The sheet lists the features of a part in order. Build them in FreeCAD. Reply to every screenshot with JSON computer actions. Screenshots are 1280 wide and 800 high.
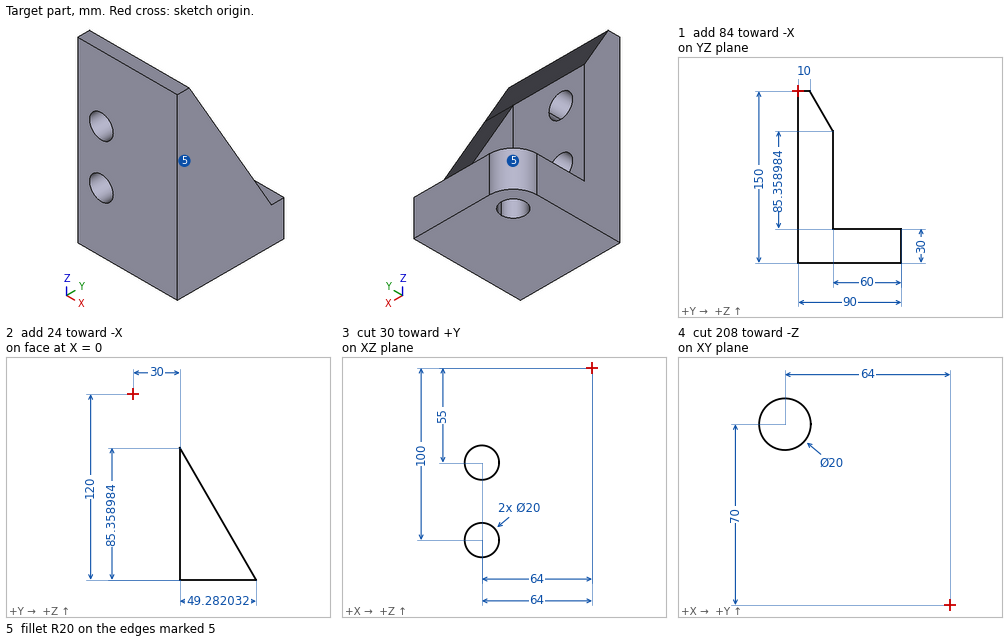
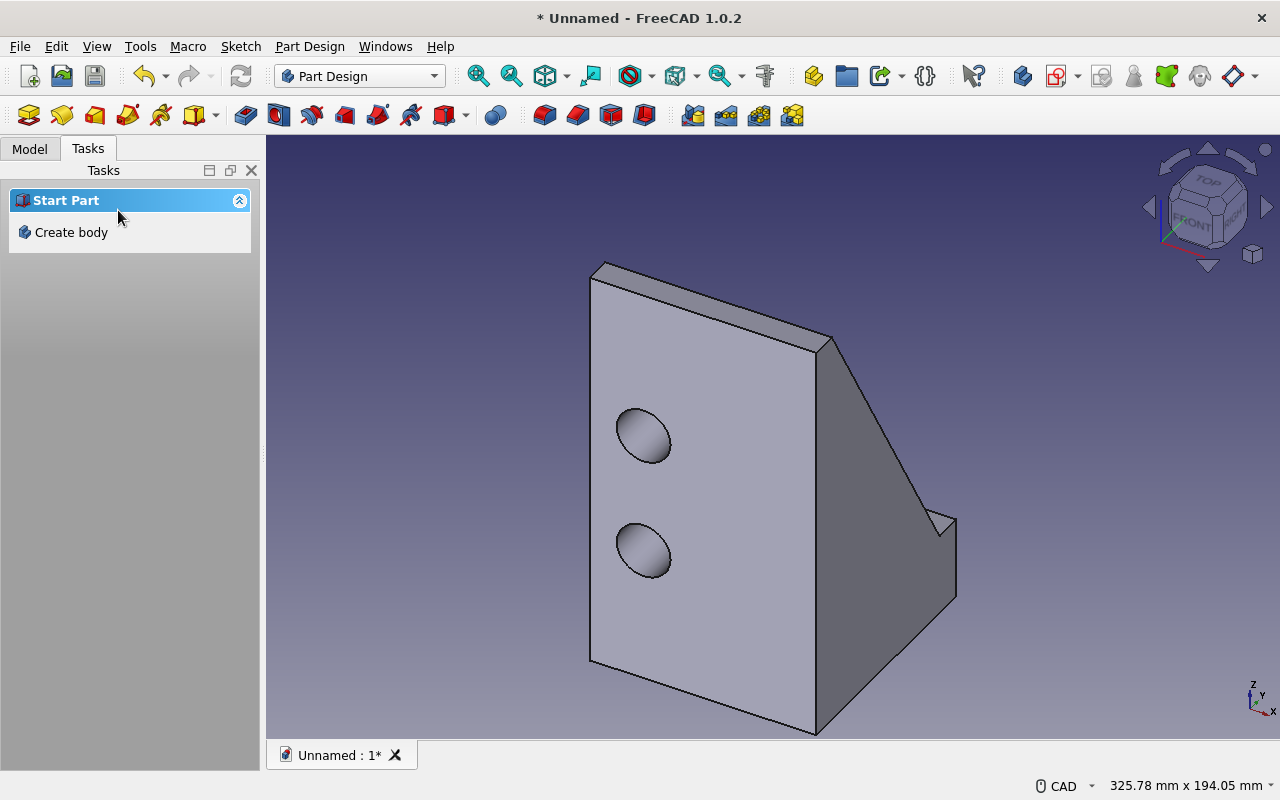
{"action": "key", "text": "0"}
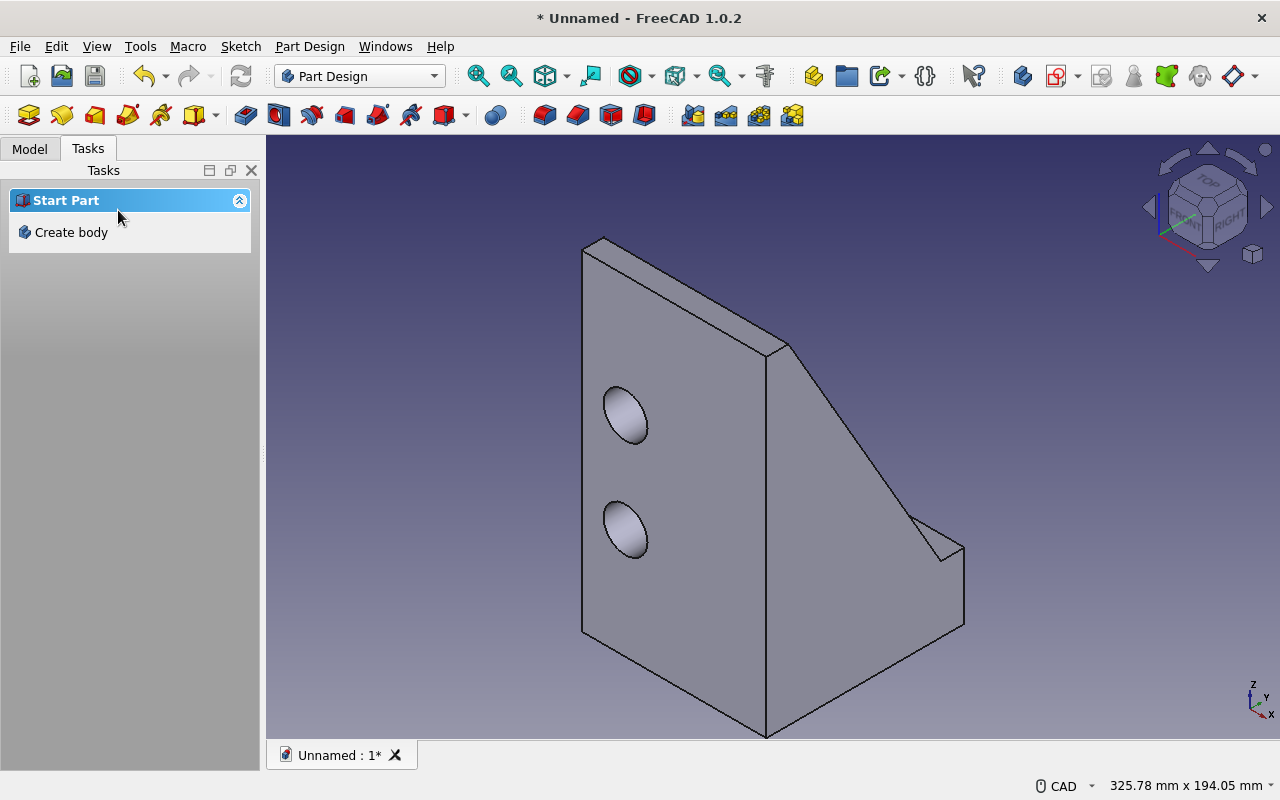
{"action": "key", "text": "2"}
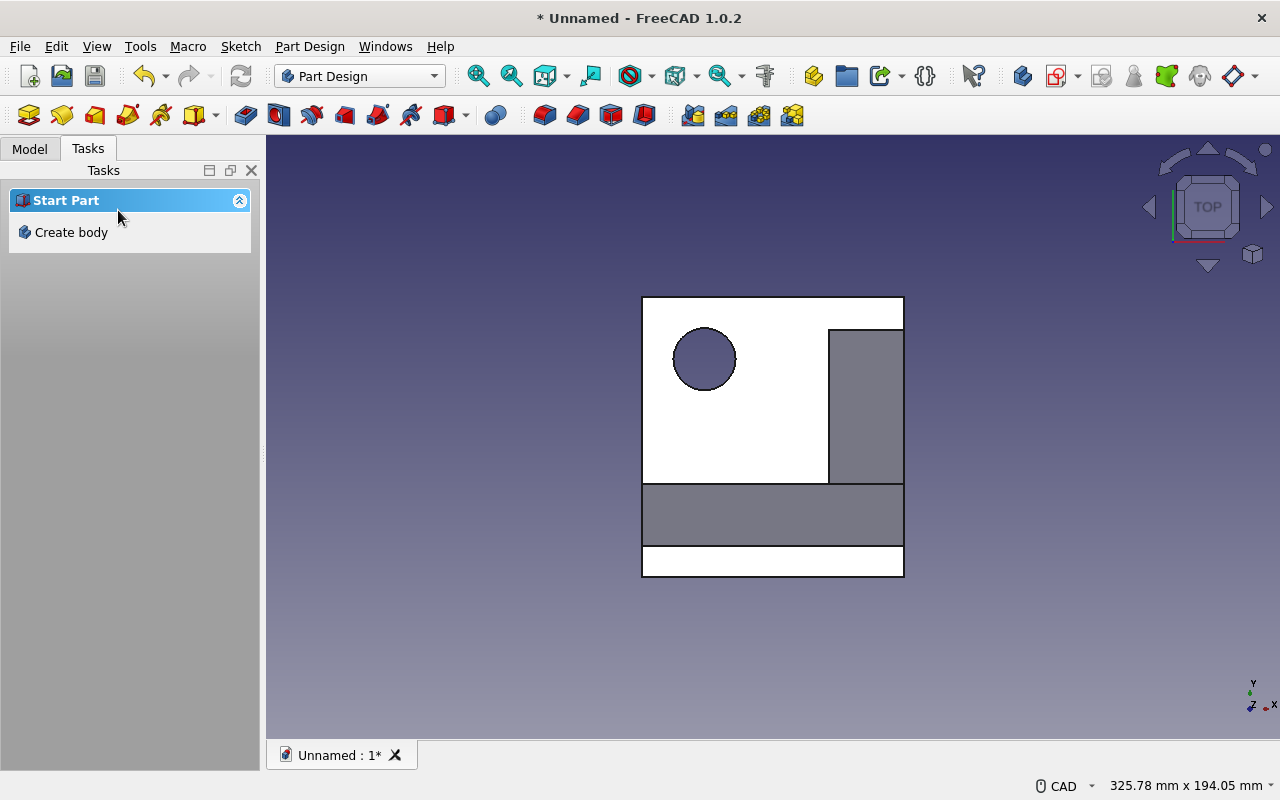
{"action": "key", "text": "1"}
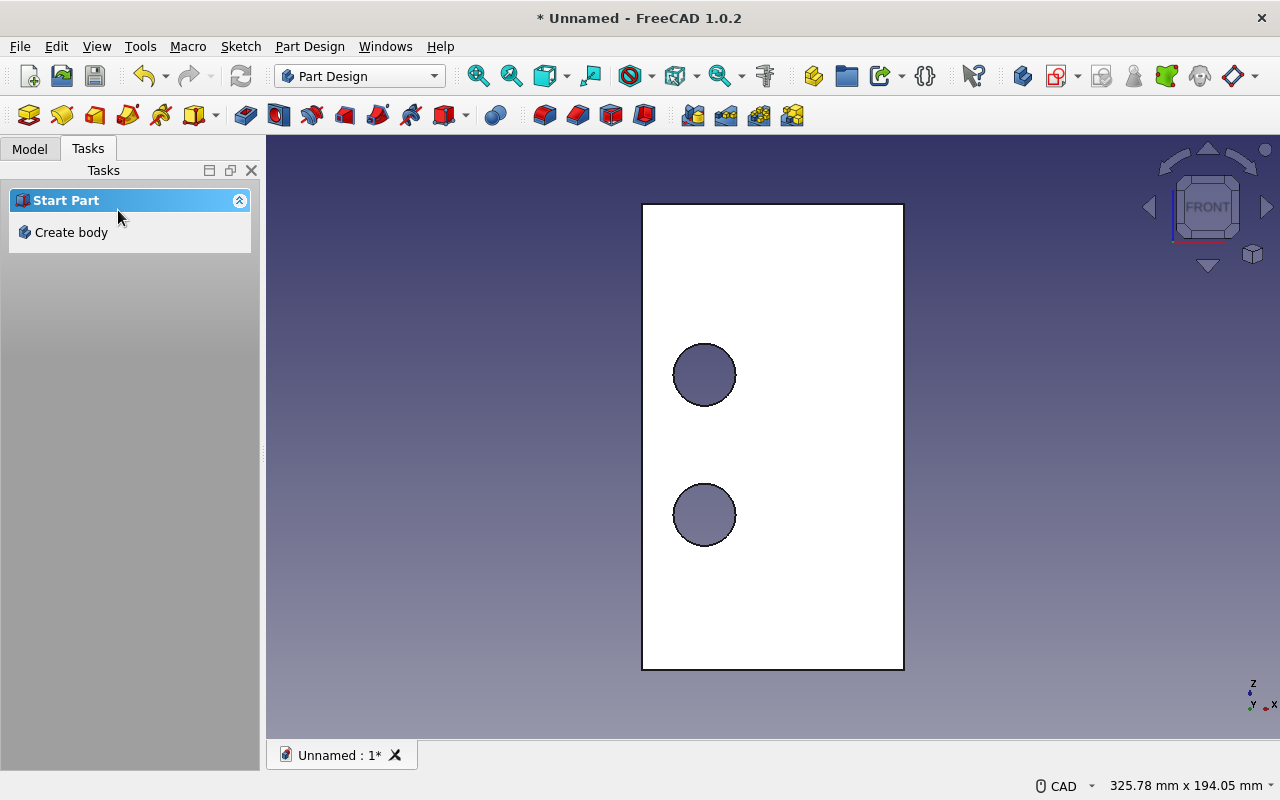
{"action": "key", "text": "3"}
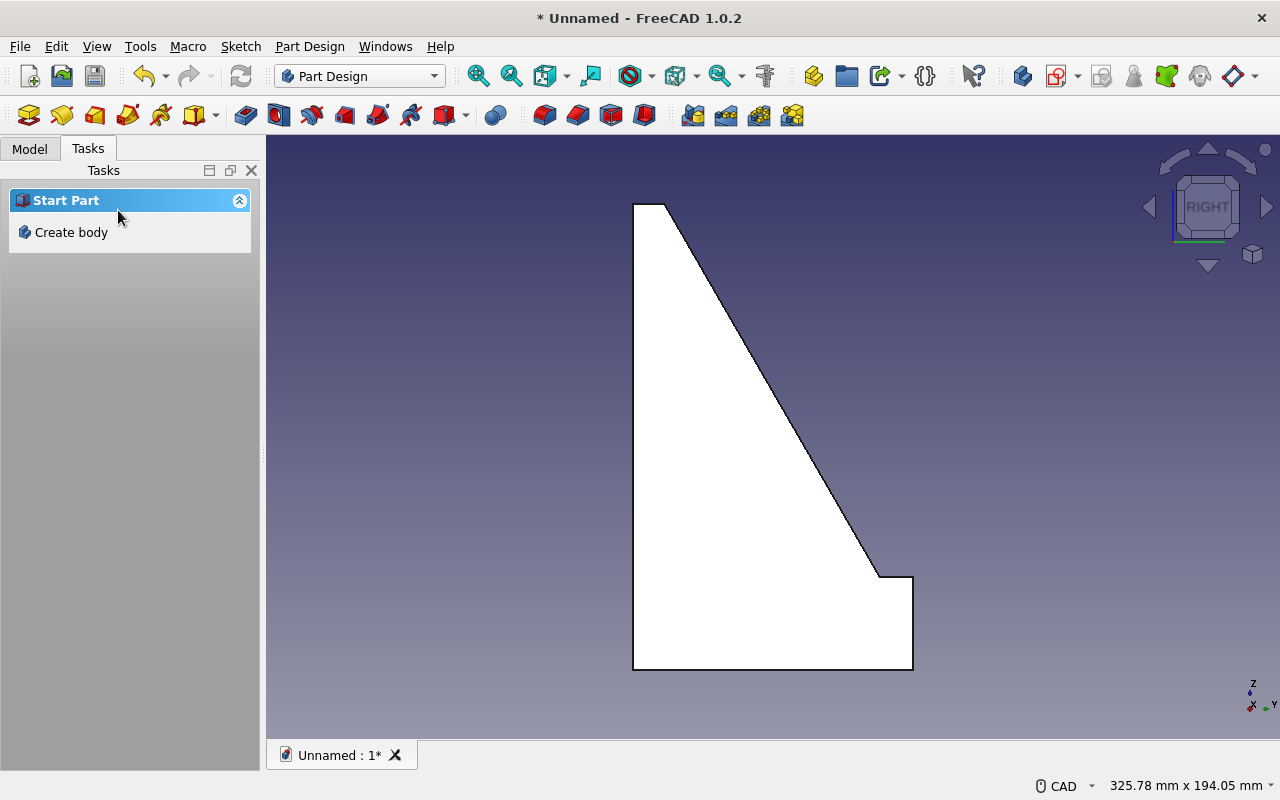
{"action": "key", "text": "5"}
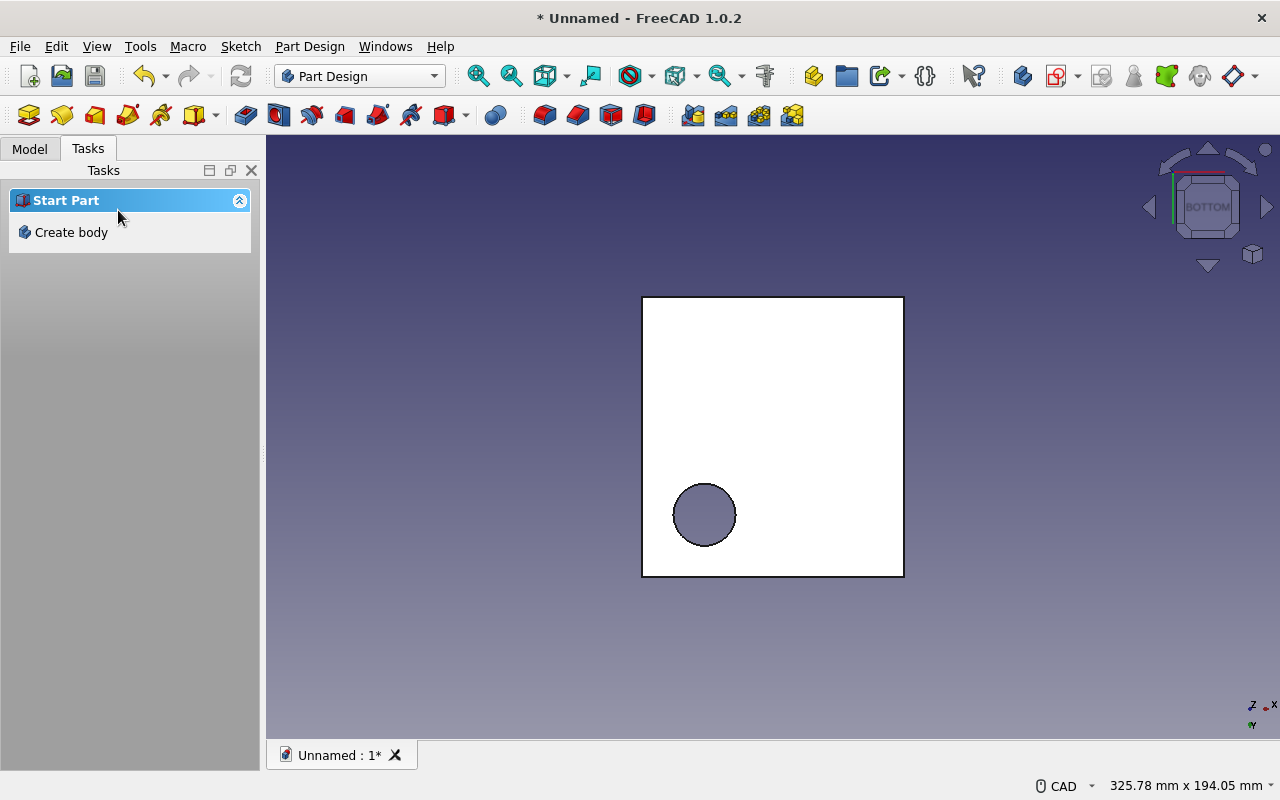
{"action": "key", "text": "4"}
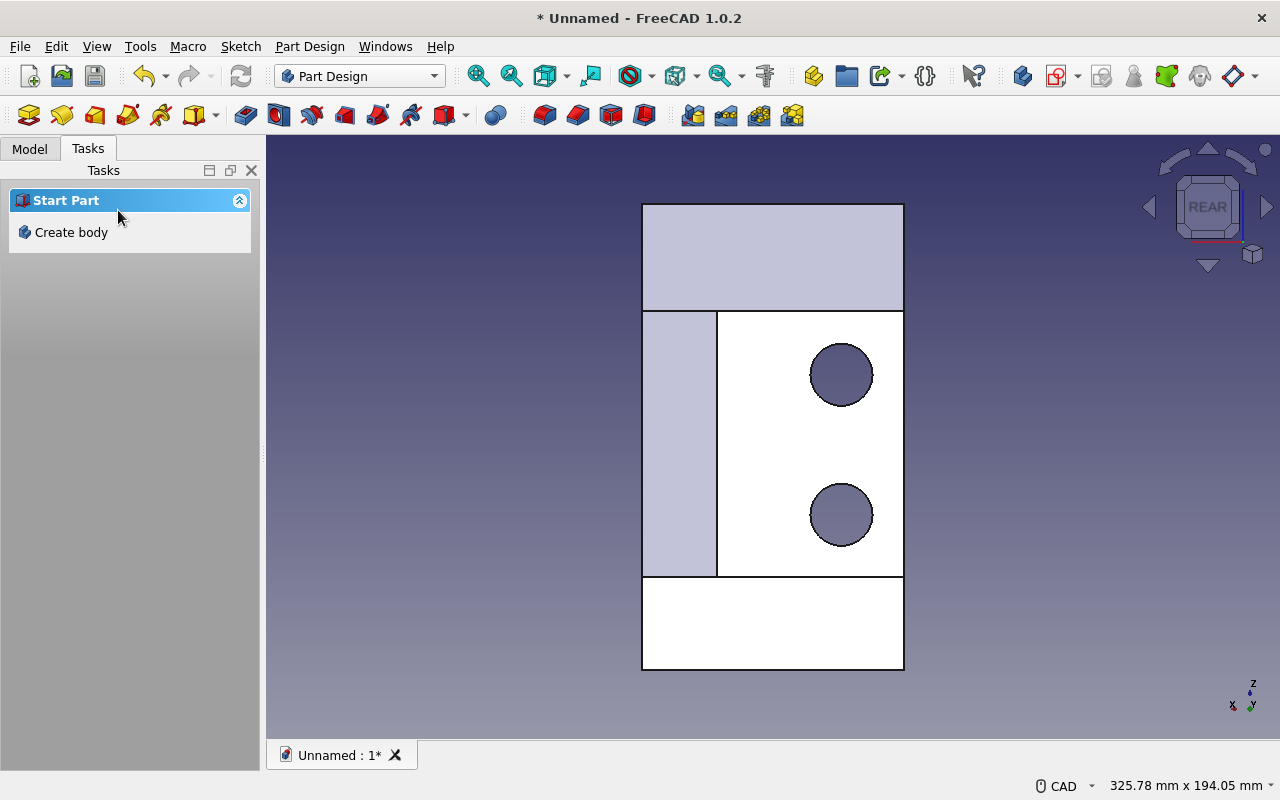
{"action": "left_click", "coordinate": [904, 623]}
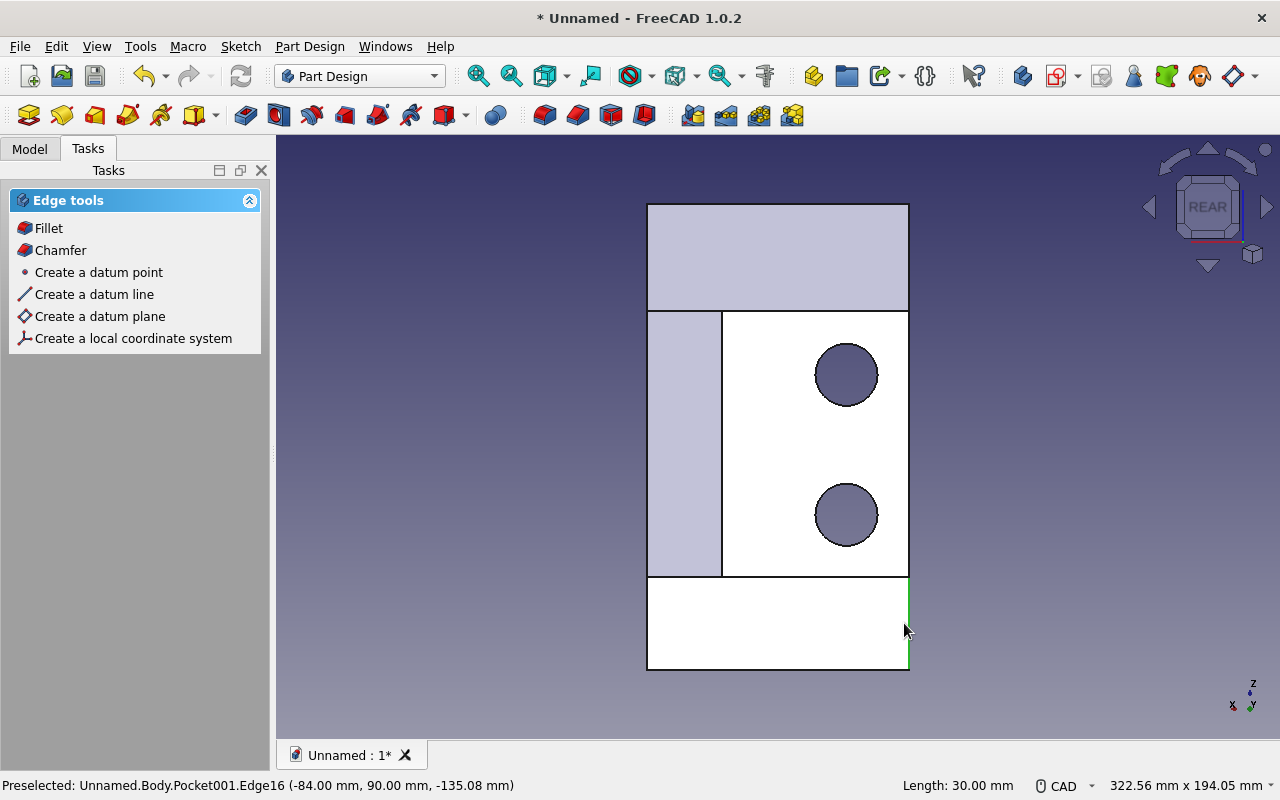
{"action": "left_click", "coordinate": [545, 116]}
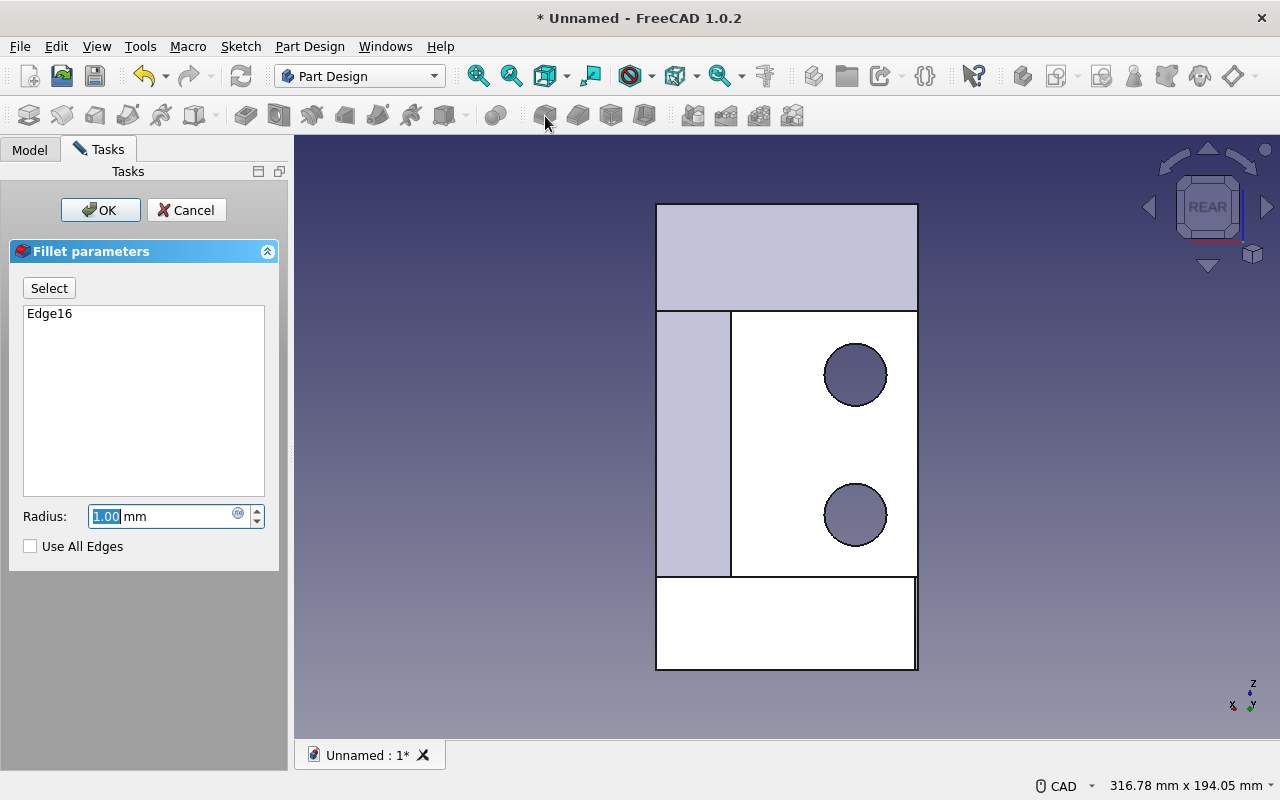
{"action": "type", "text": "20"}
{"action": "key", "text": "Tab"}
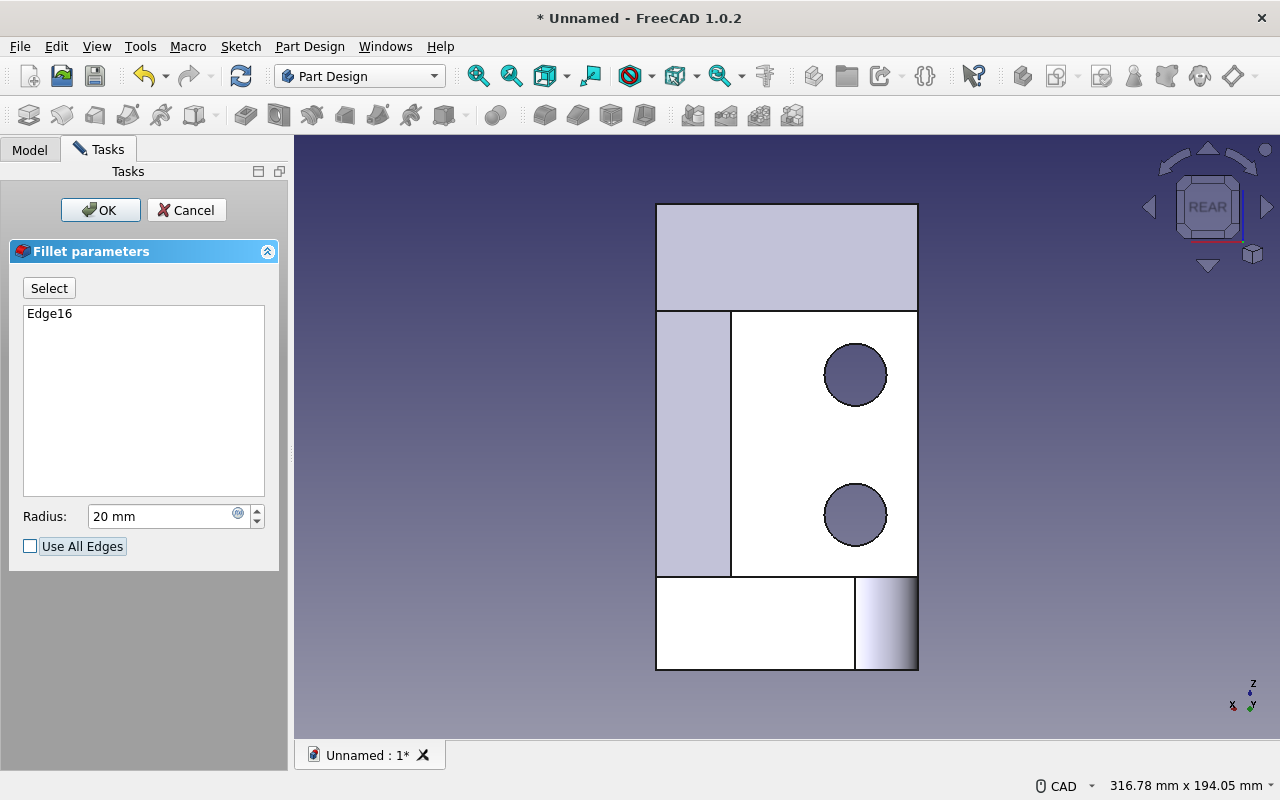
{"action": "left_click", "coordinate": [101, 210]}